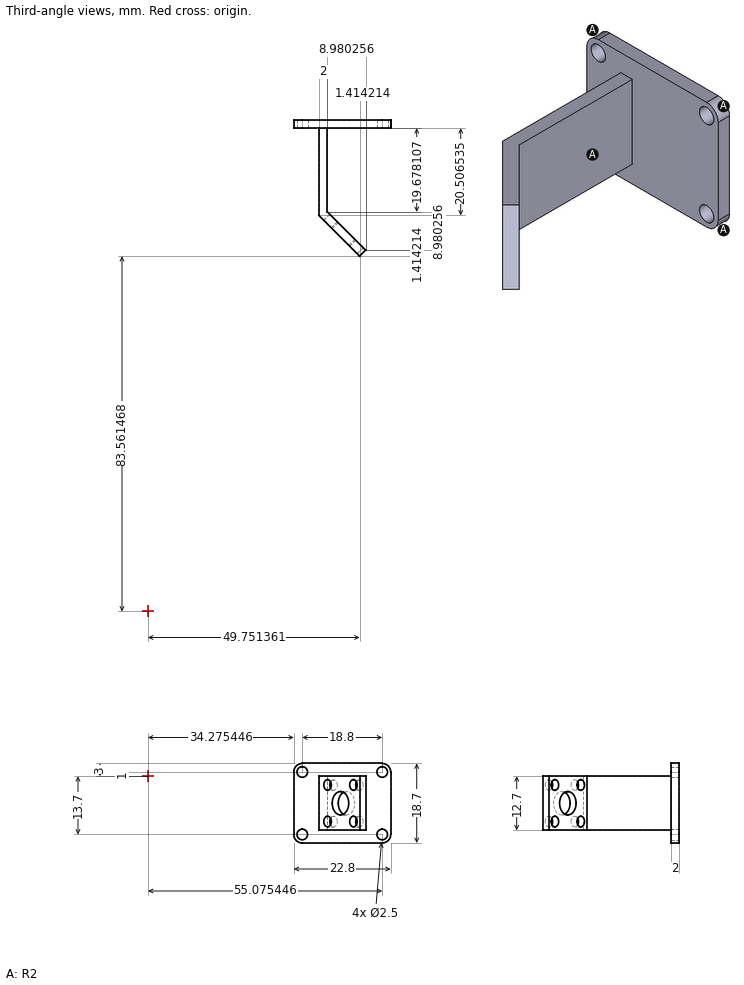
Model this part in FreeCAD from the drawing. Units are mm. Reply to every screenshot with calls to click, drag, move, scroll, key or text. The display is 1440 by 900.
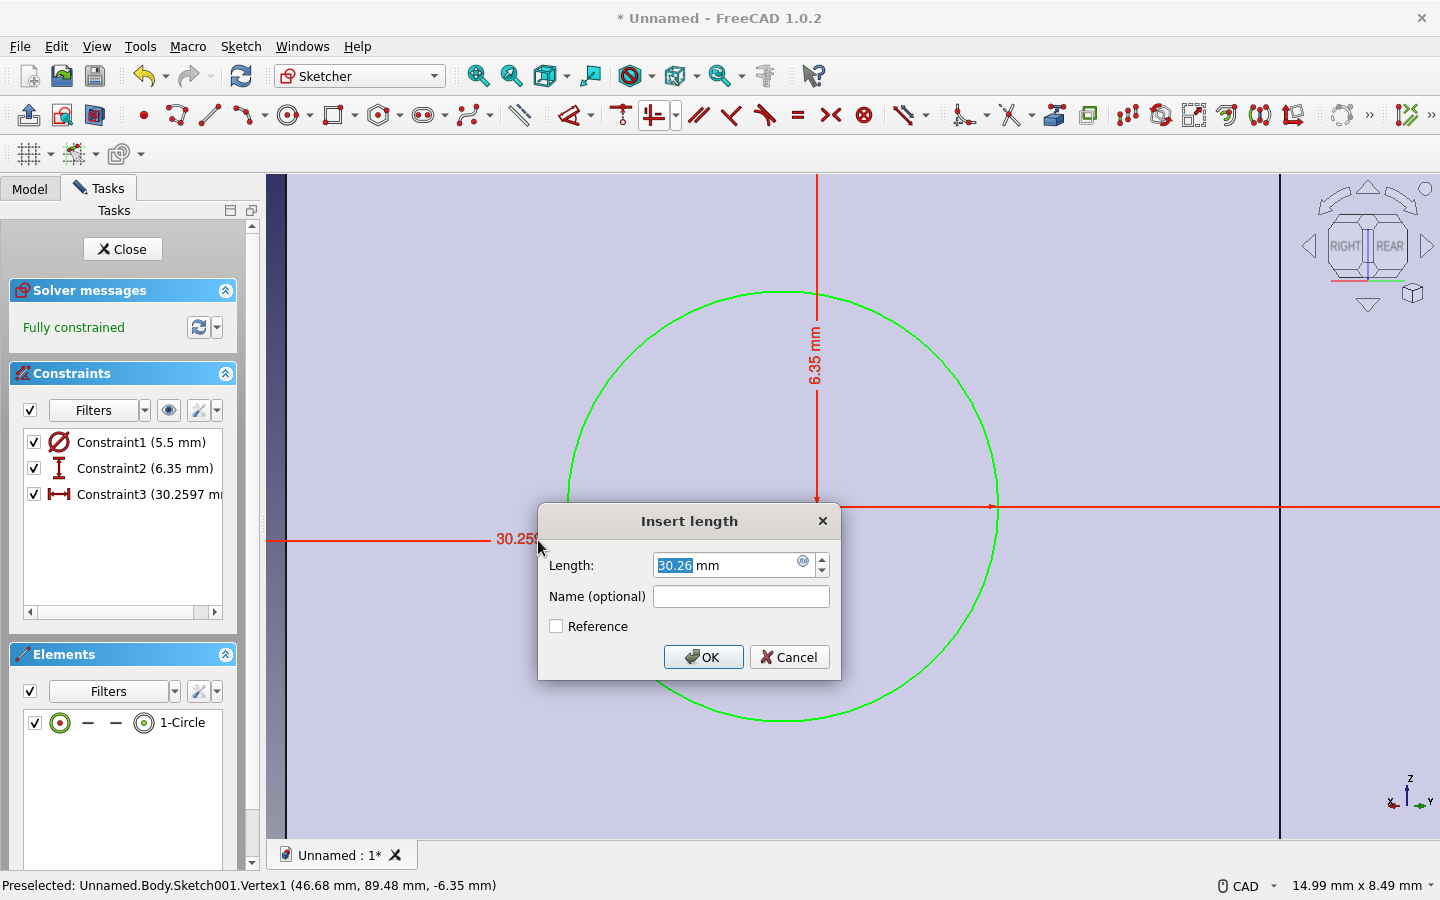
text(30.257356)
key(Return)
key(Escape)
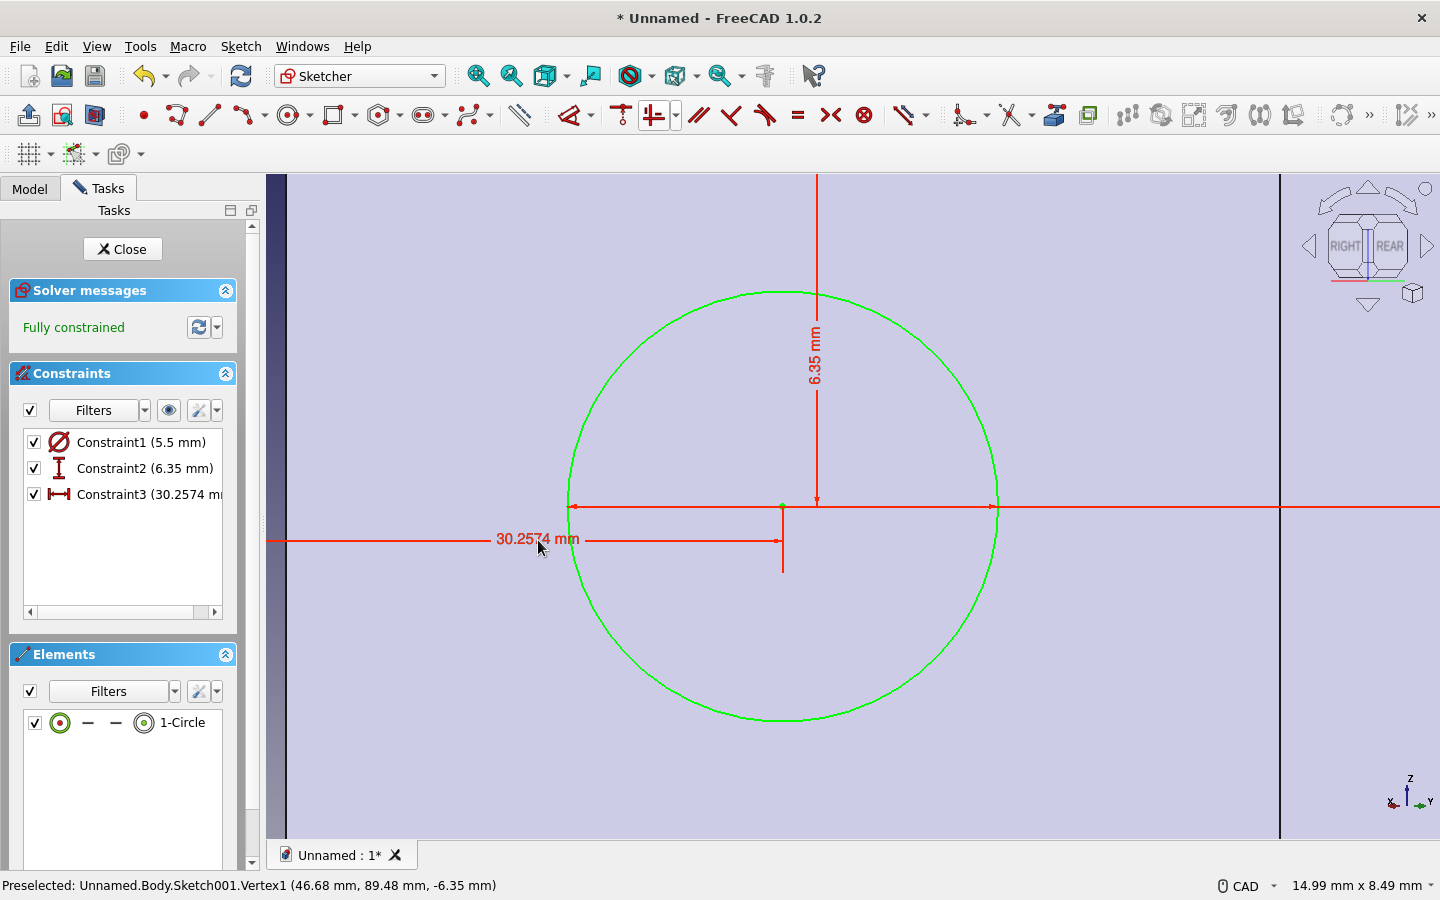
click(123, 249)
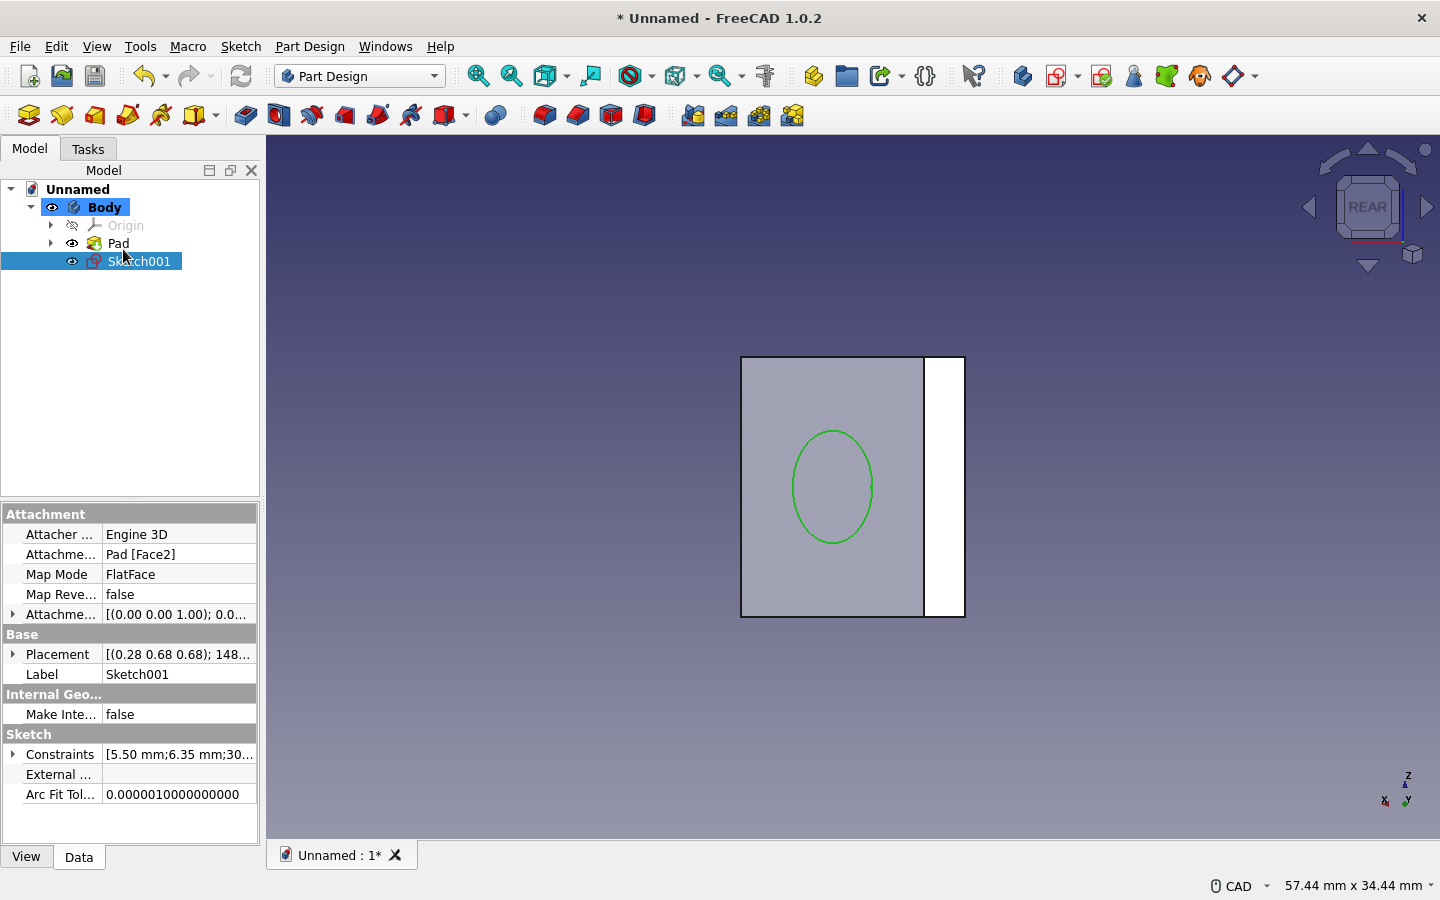
click(246, 116)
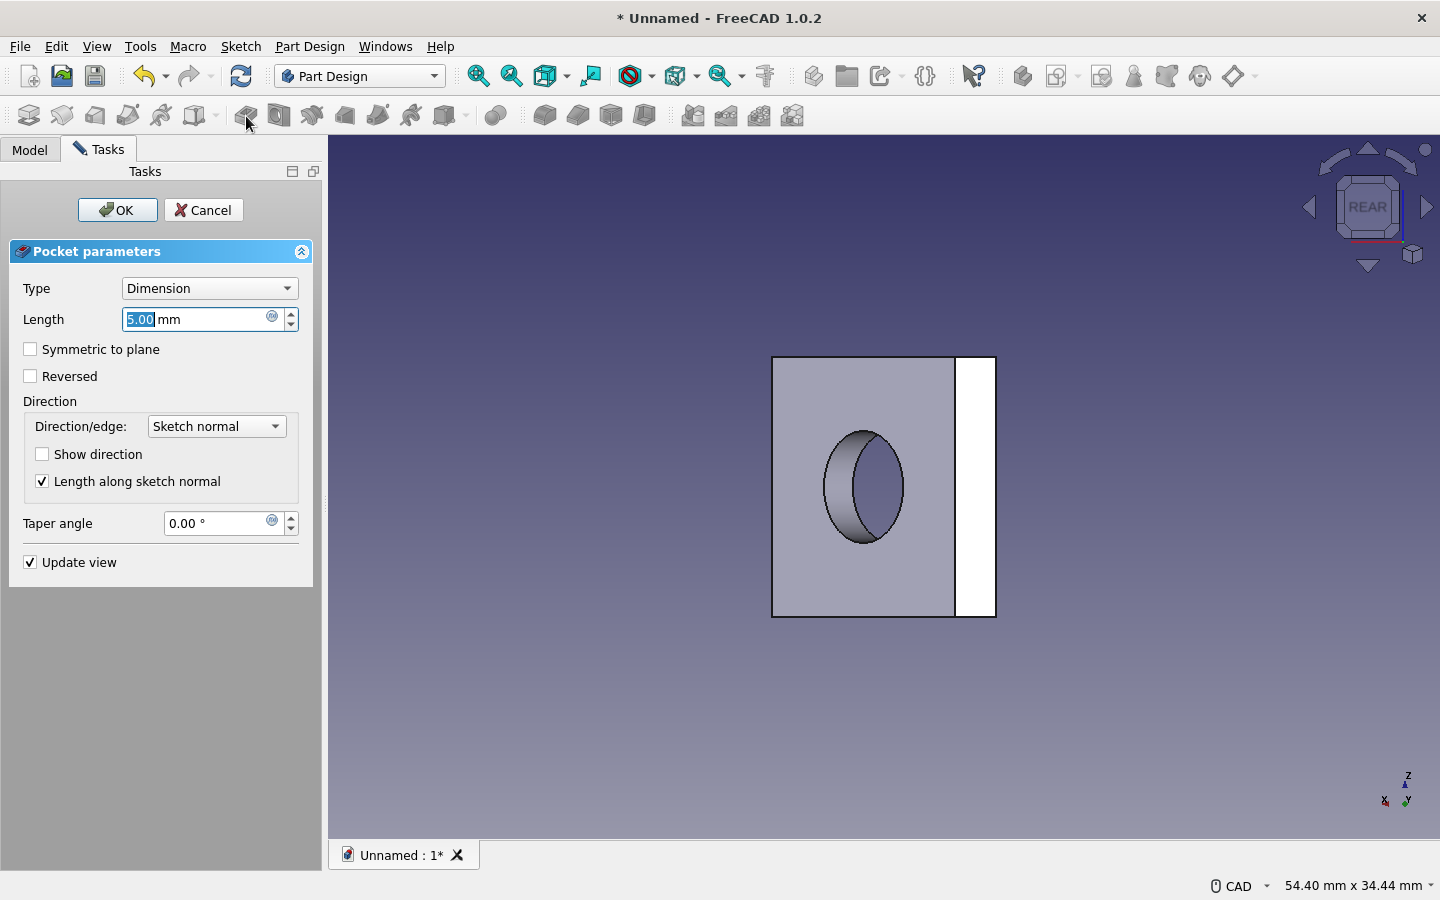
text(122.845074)
key(Tab)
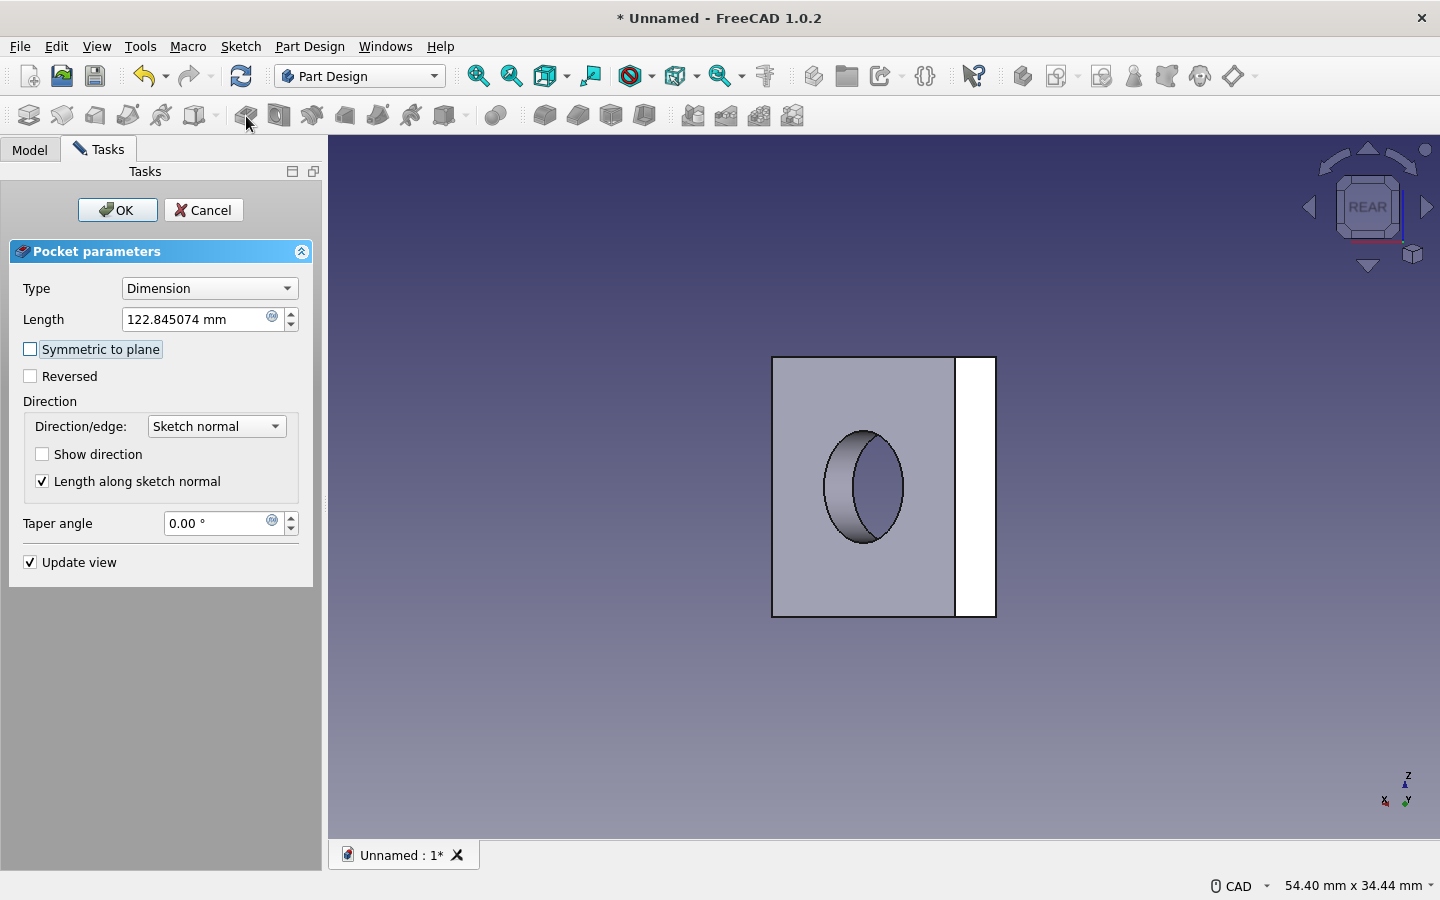
click(31, 349)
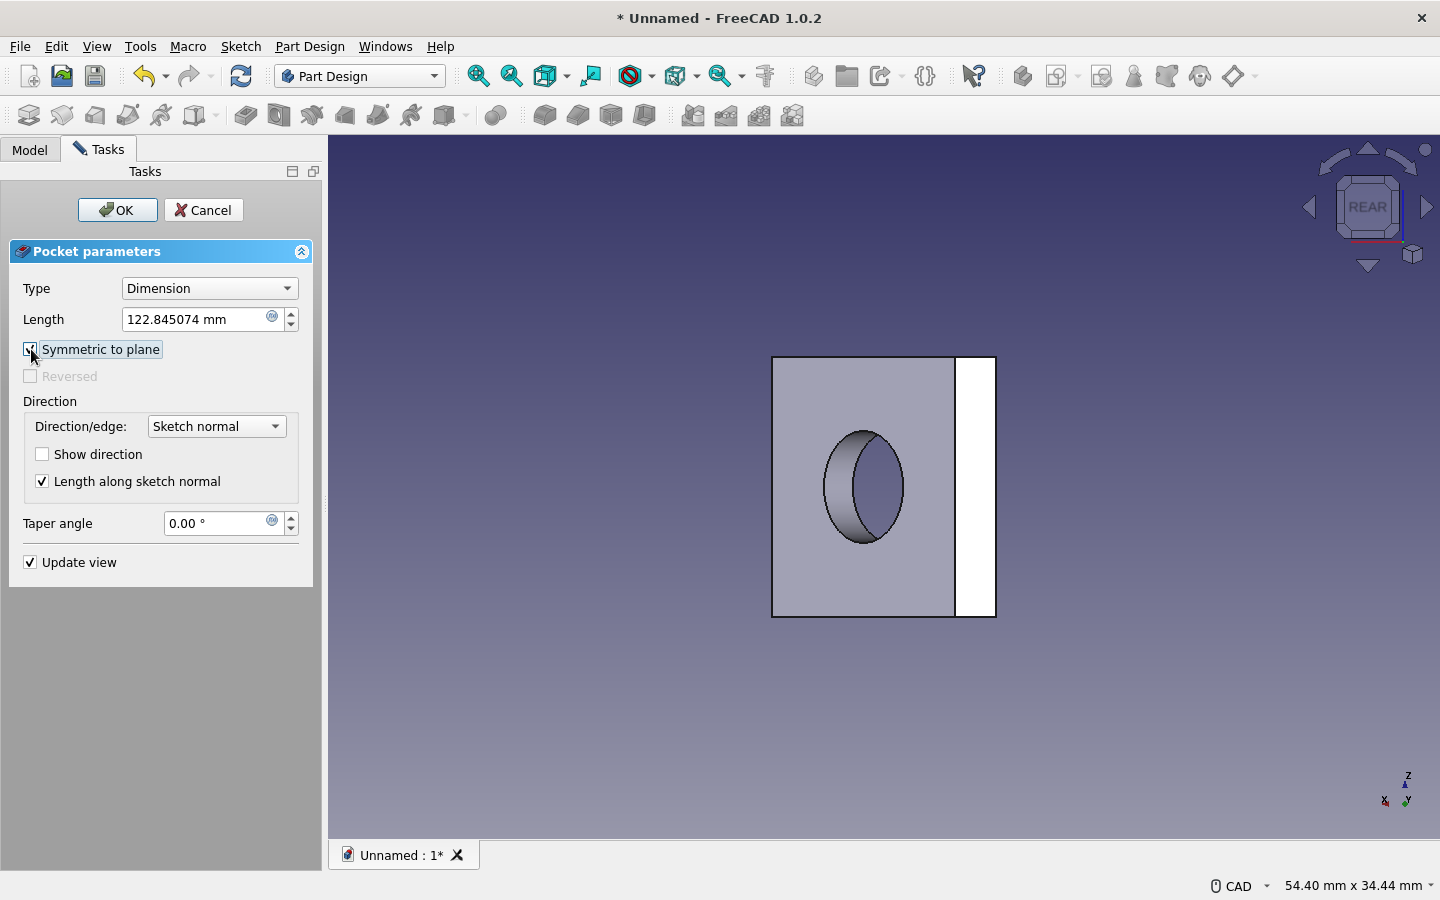
click(118, 210)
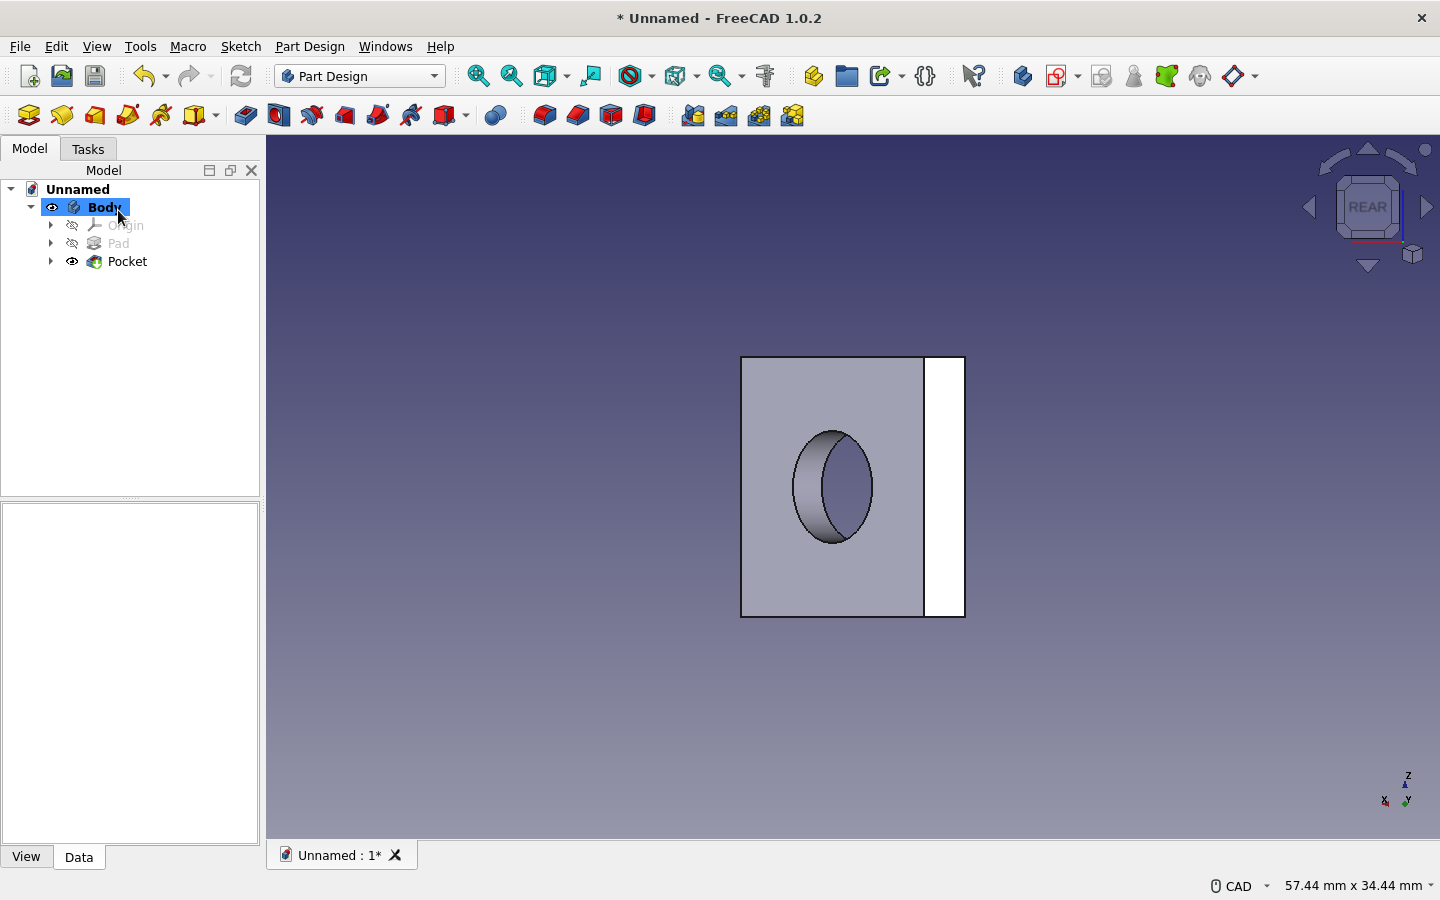
click(479, 76)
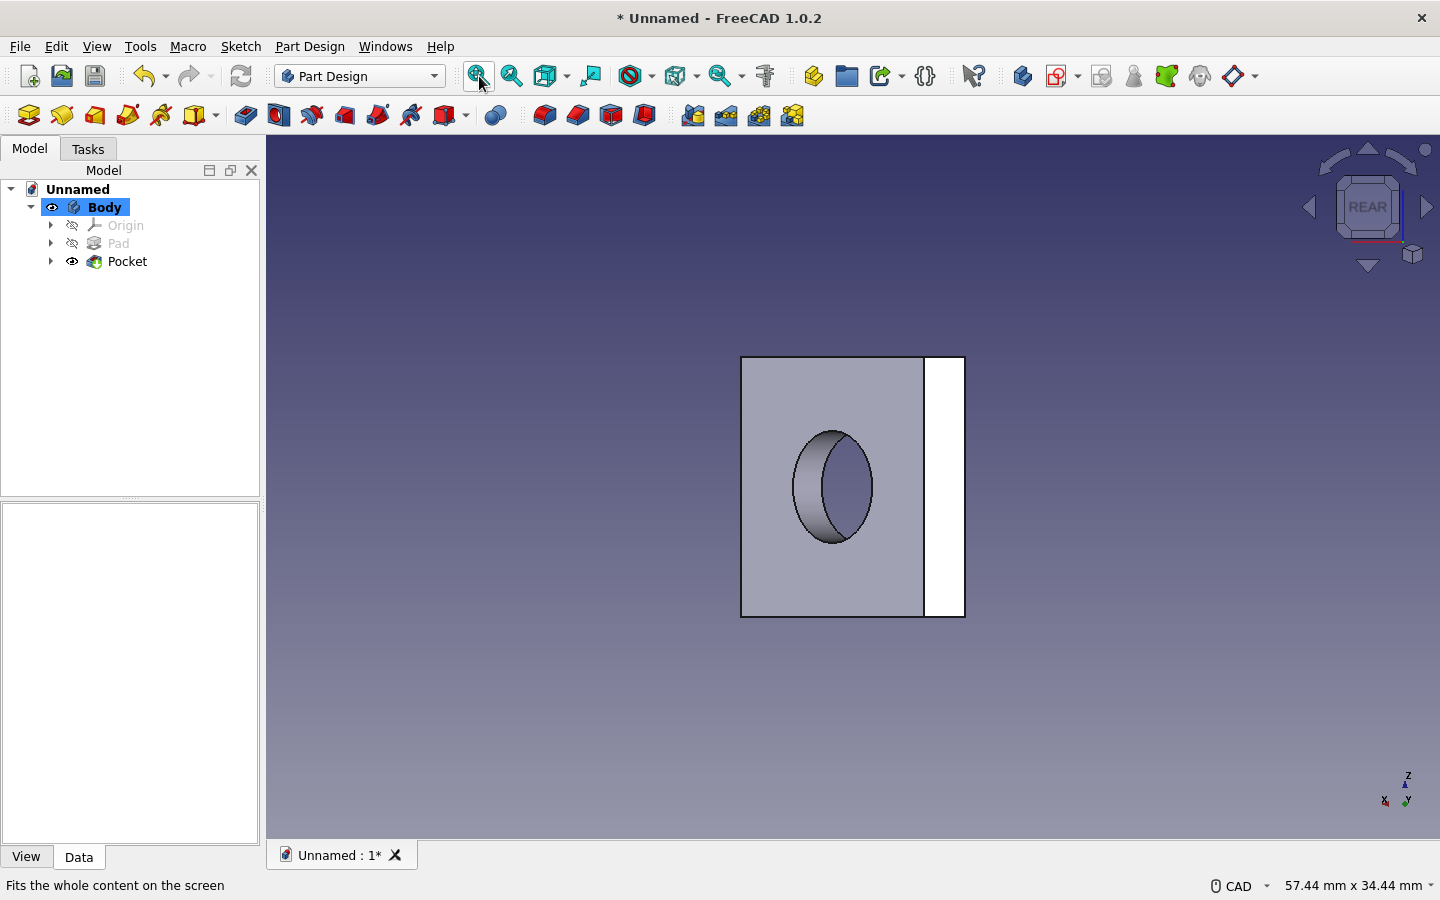
key(1)